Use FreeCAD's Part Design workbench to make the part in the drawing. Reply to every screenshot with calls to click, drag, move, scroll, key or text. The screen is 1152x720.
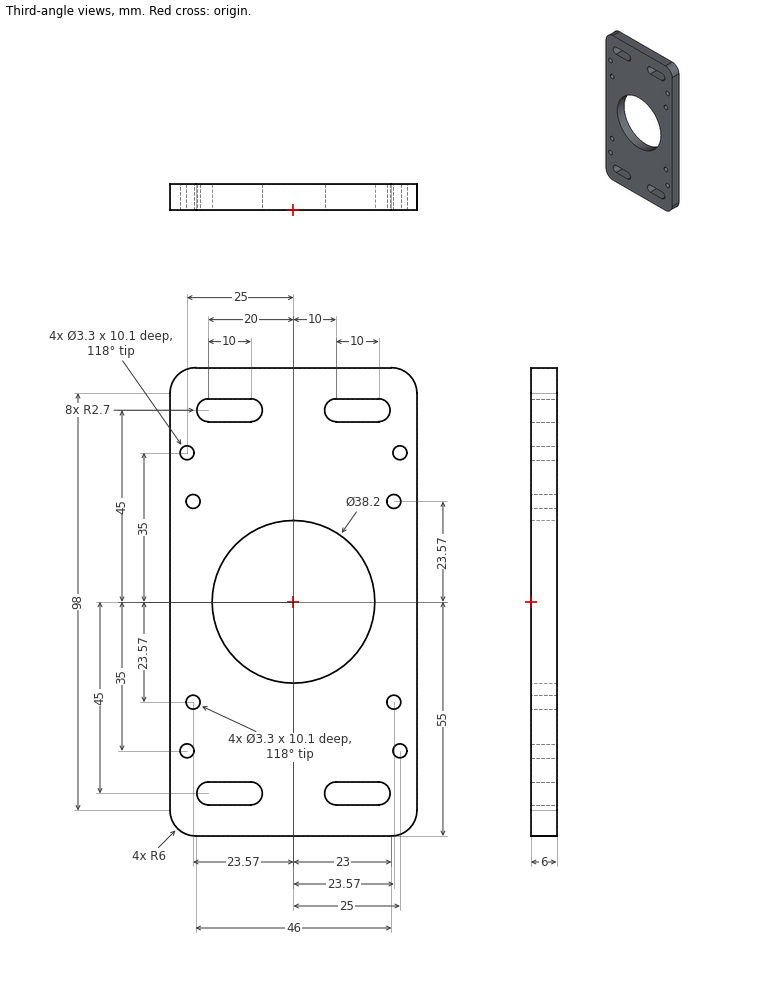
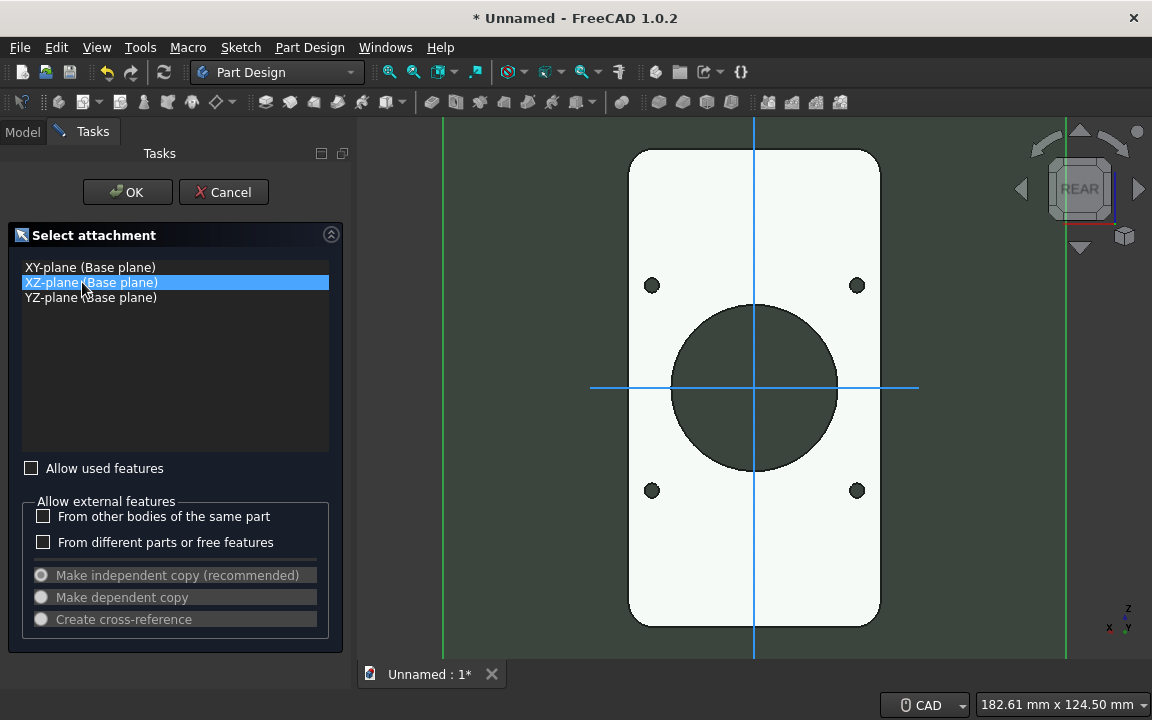
click(128, 192)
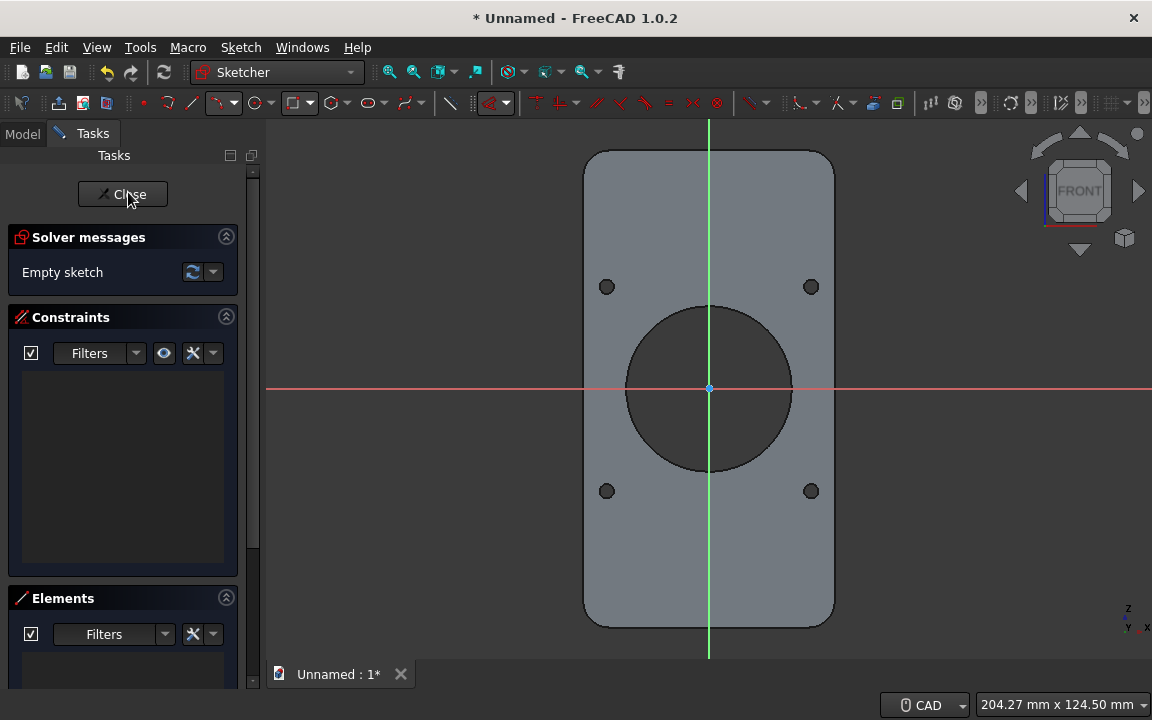
key(g)
key(s)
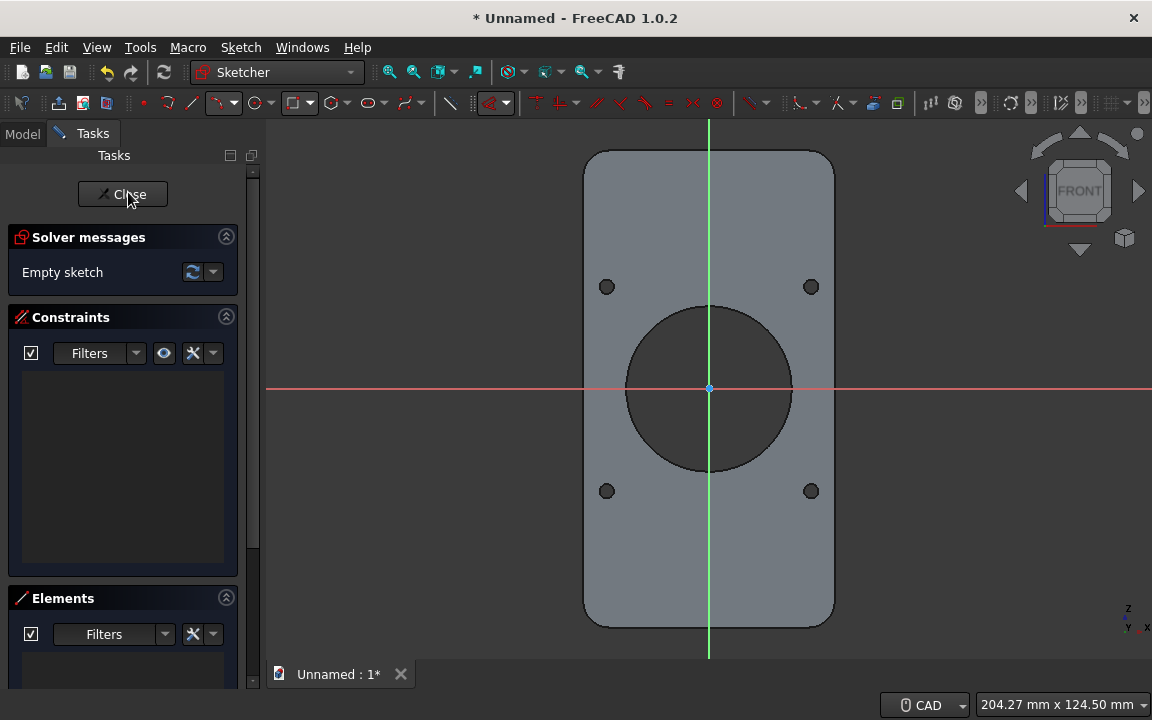
scroll(622, 194, up, 4)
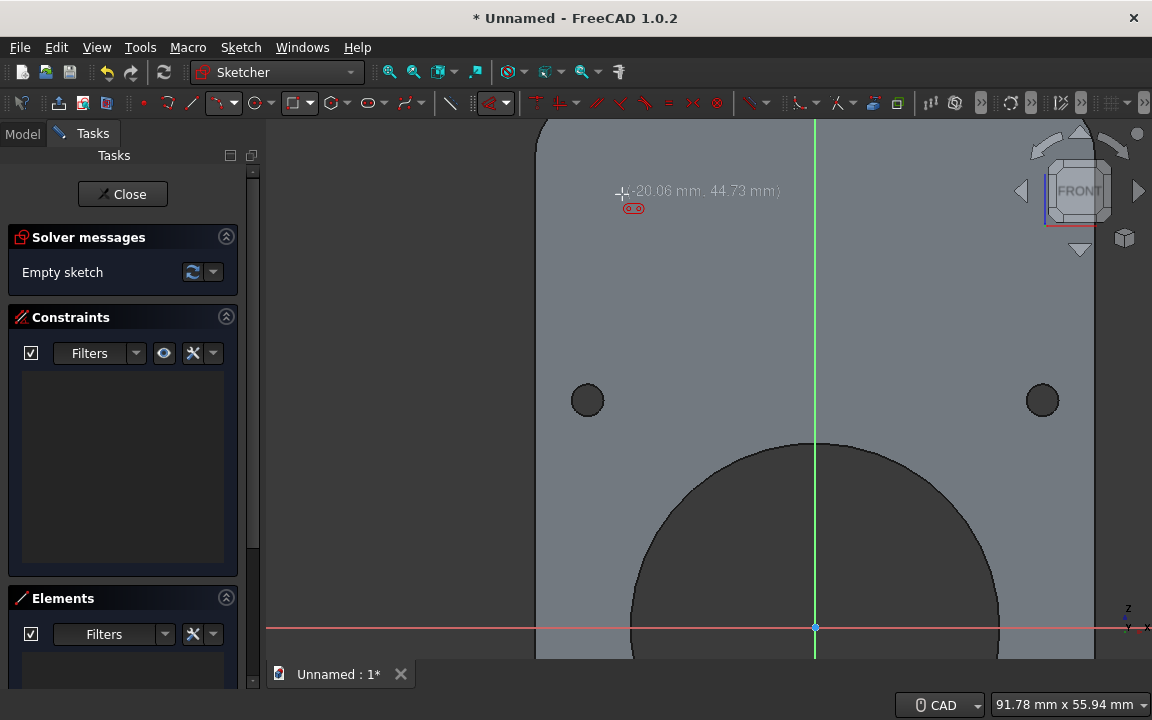
click(622, 193)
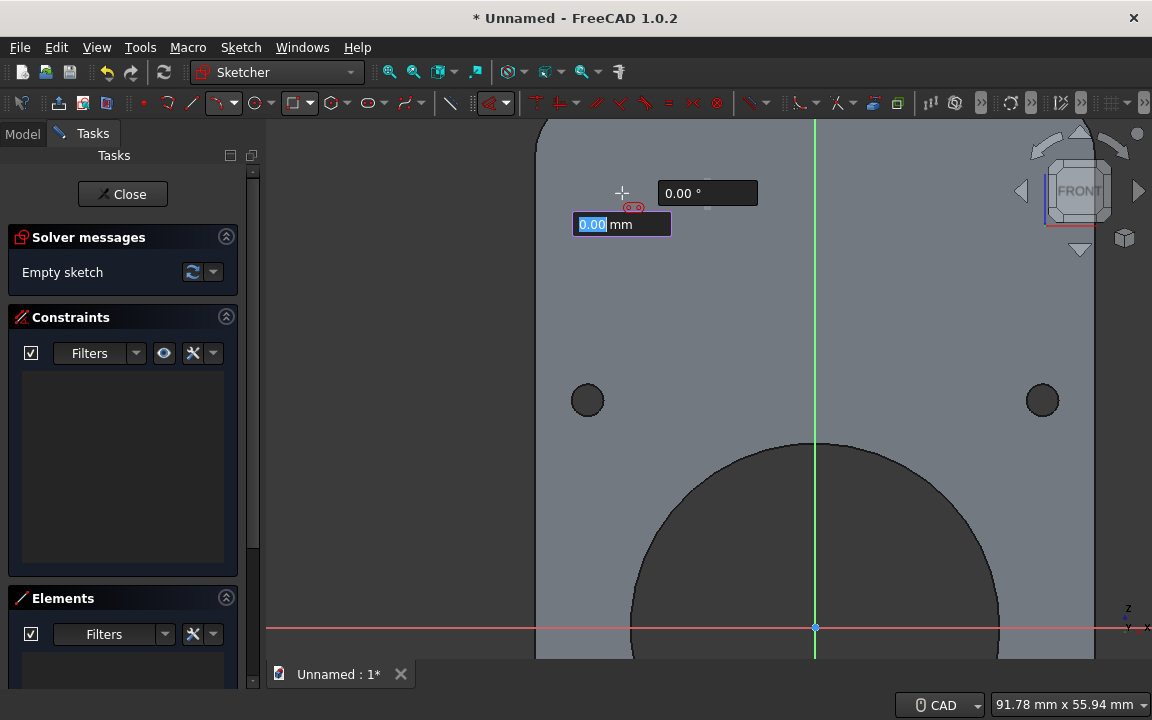
click(719, 193)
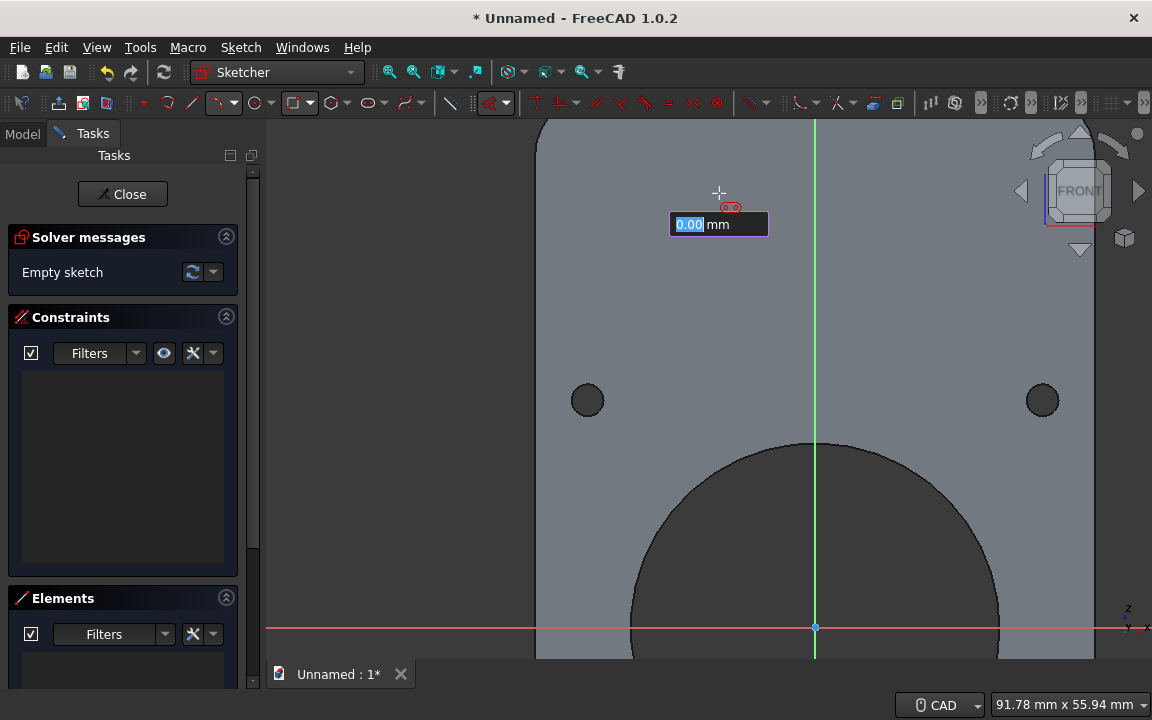
click(670, 167)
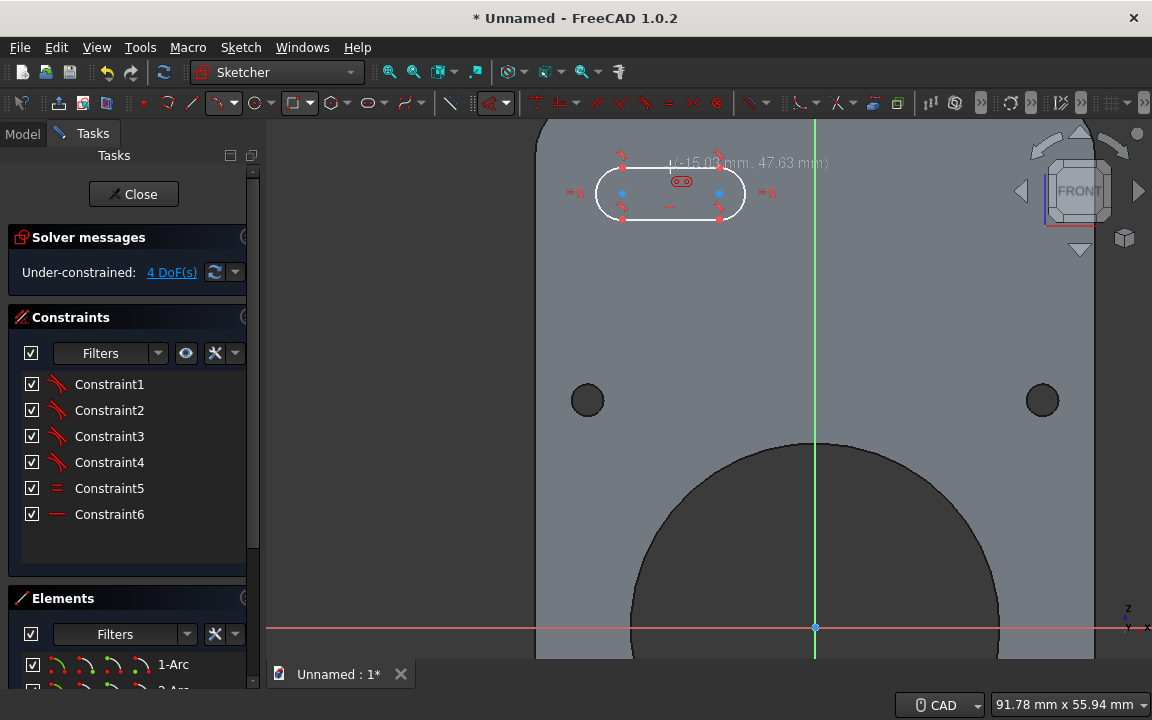
click(912, 193)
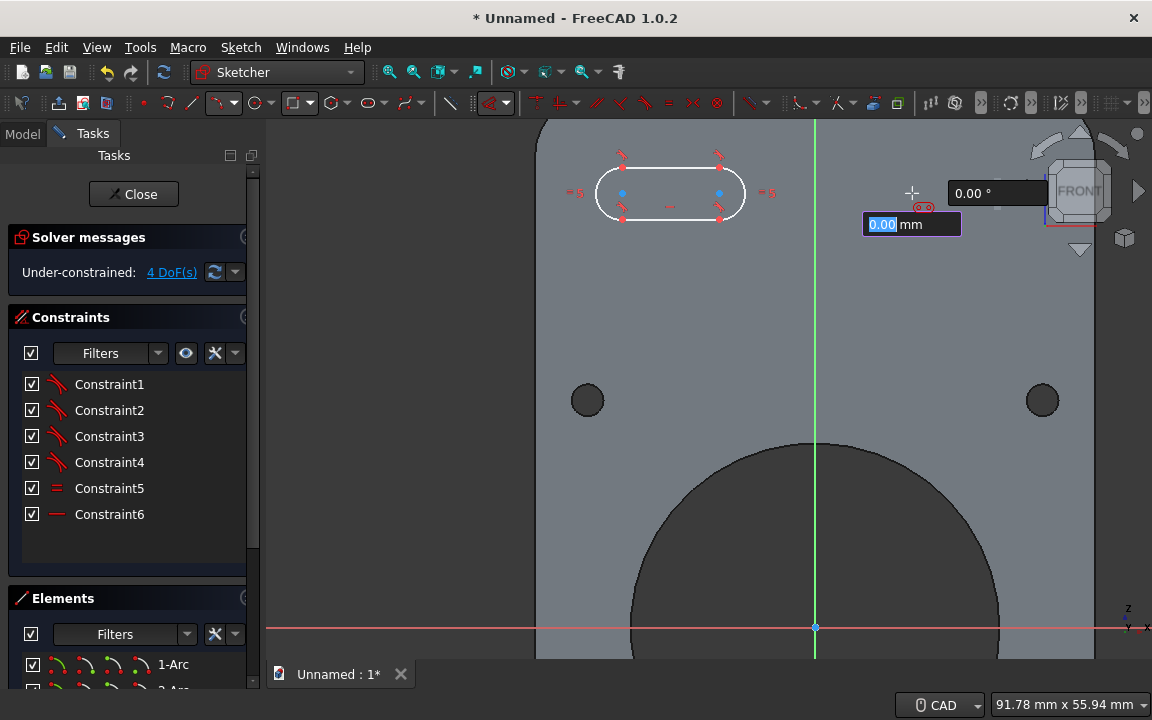
scroll(539, 250, down, 5)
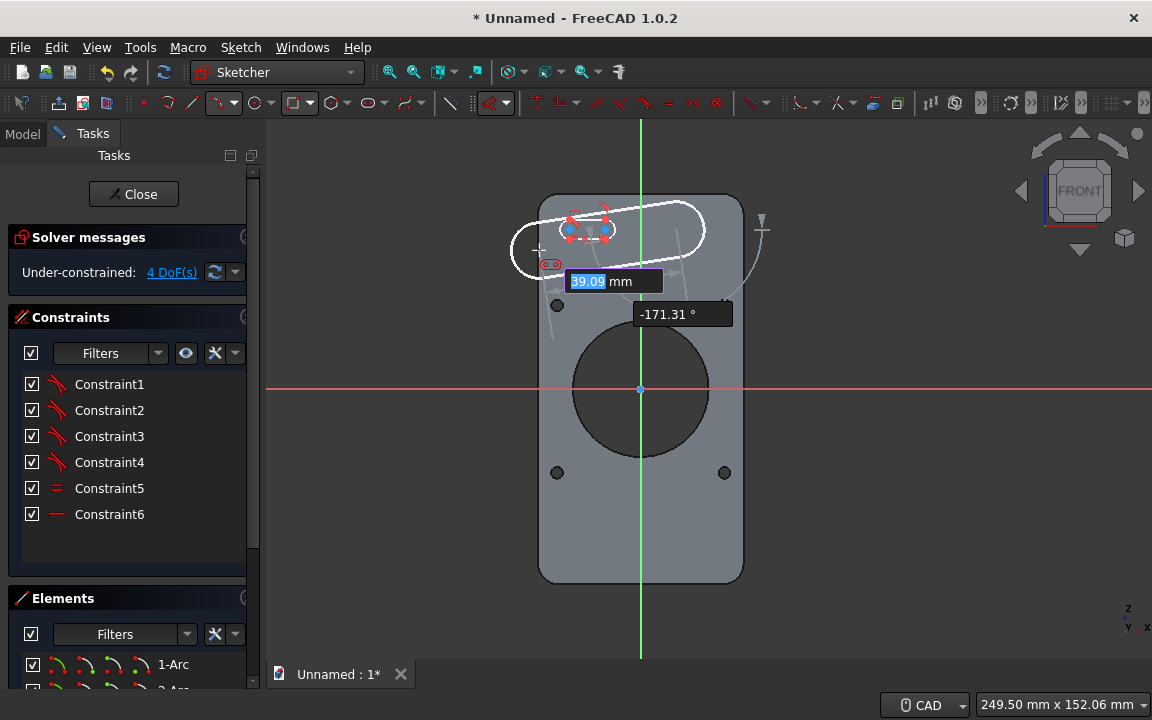
click(712, 229)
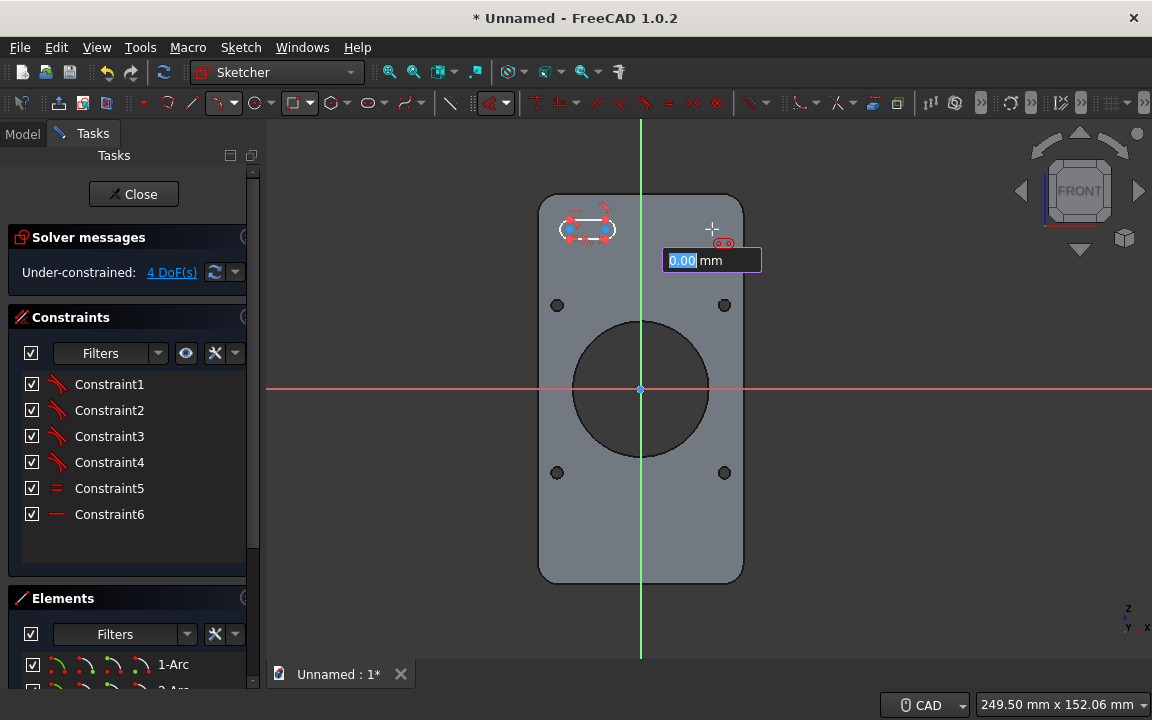
scroll(694, 220, up, 3)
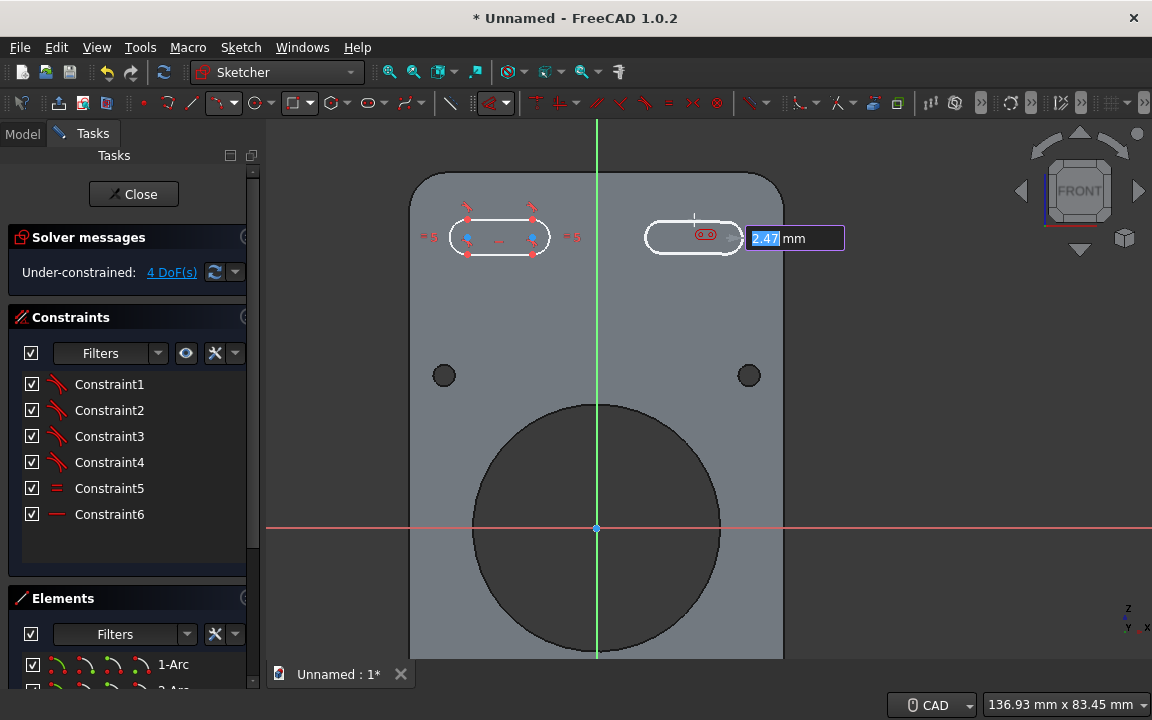
click(694, 219)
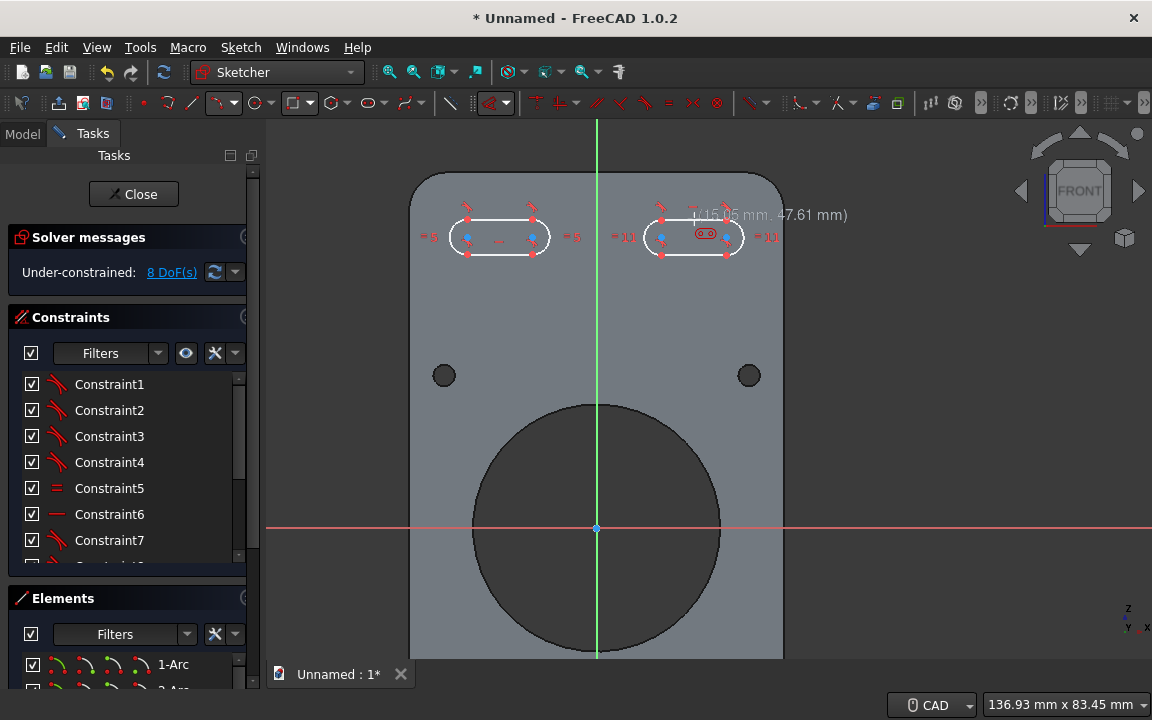
scroll(694, 220, down, 3)